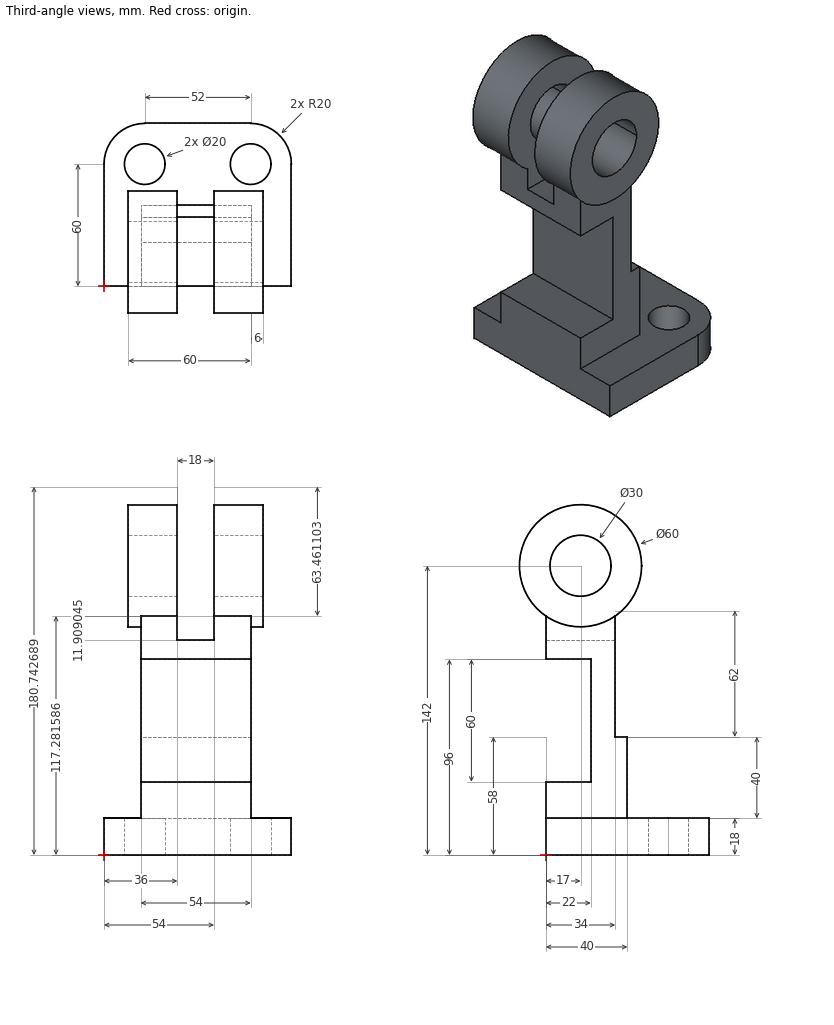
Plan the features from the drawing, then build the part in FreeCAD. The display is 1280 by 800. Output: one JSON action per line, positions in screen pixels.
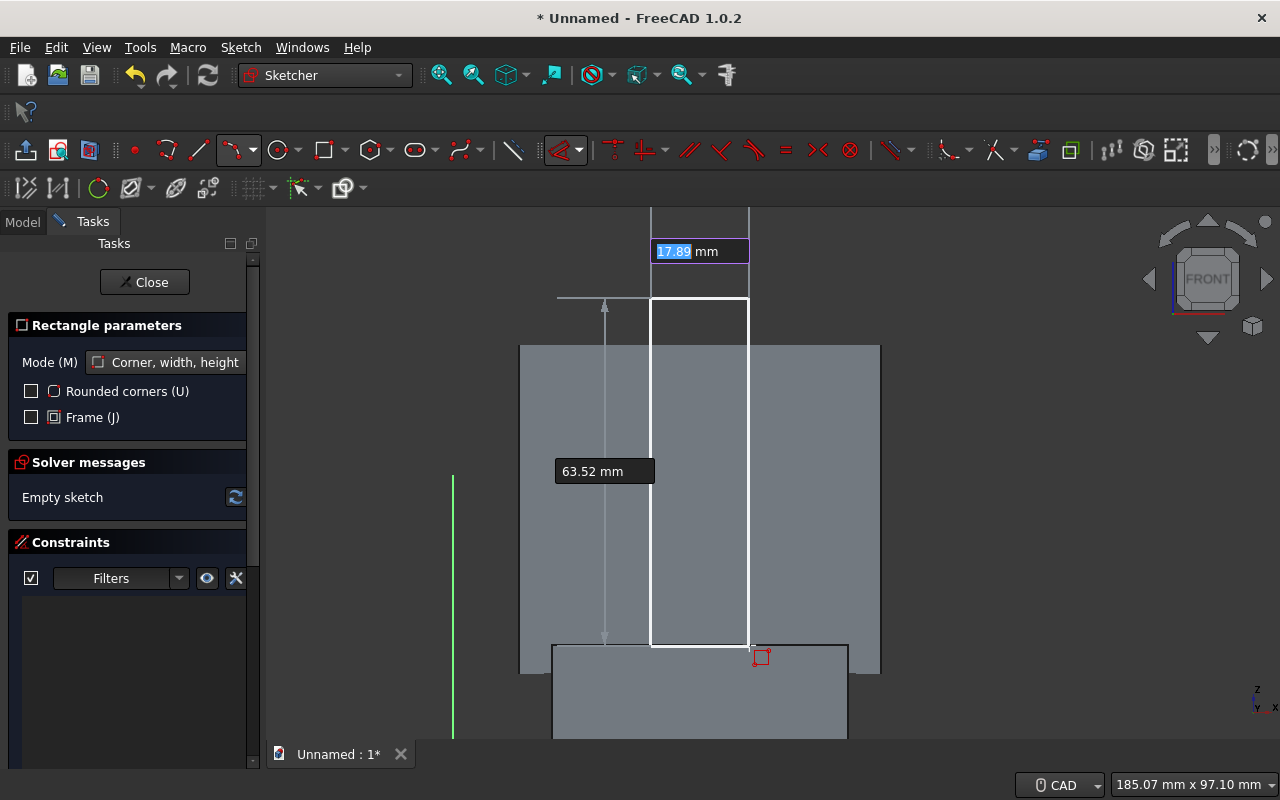
{"action": "type", "text": "18"}
{"action": "key", "text": "Tab"}
{"action": "type", "text": "63.461103"}
{"action": "key", "text": "Return"}
{"action": "key", "text": "Escape"}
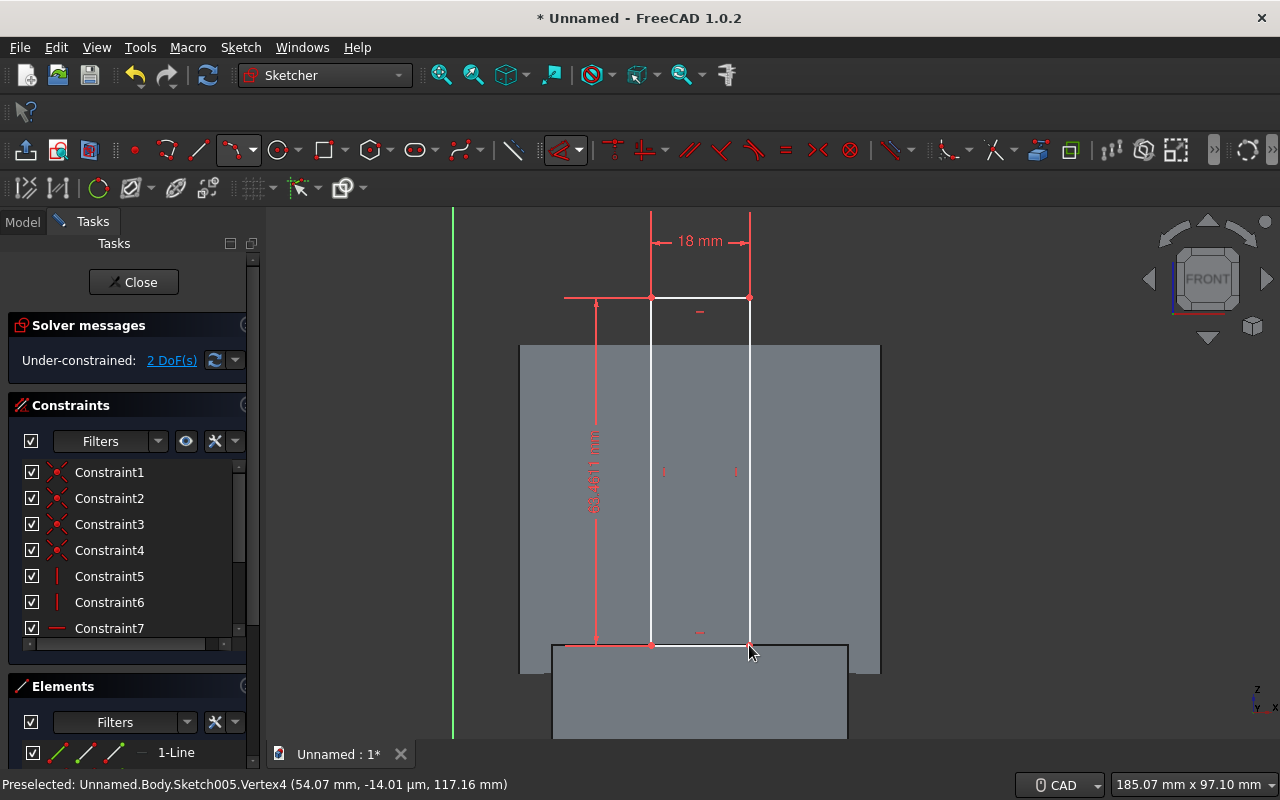
{"action": "left_click", "coordinate": [651, 298]}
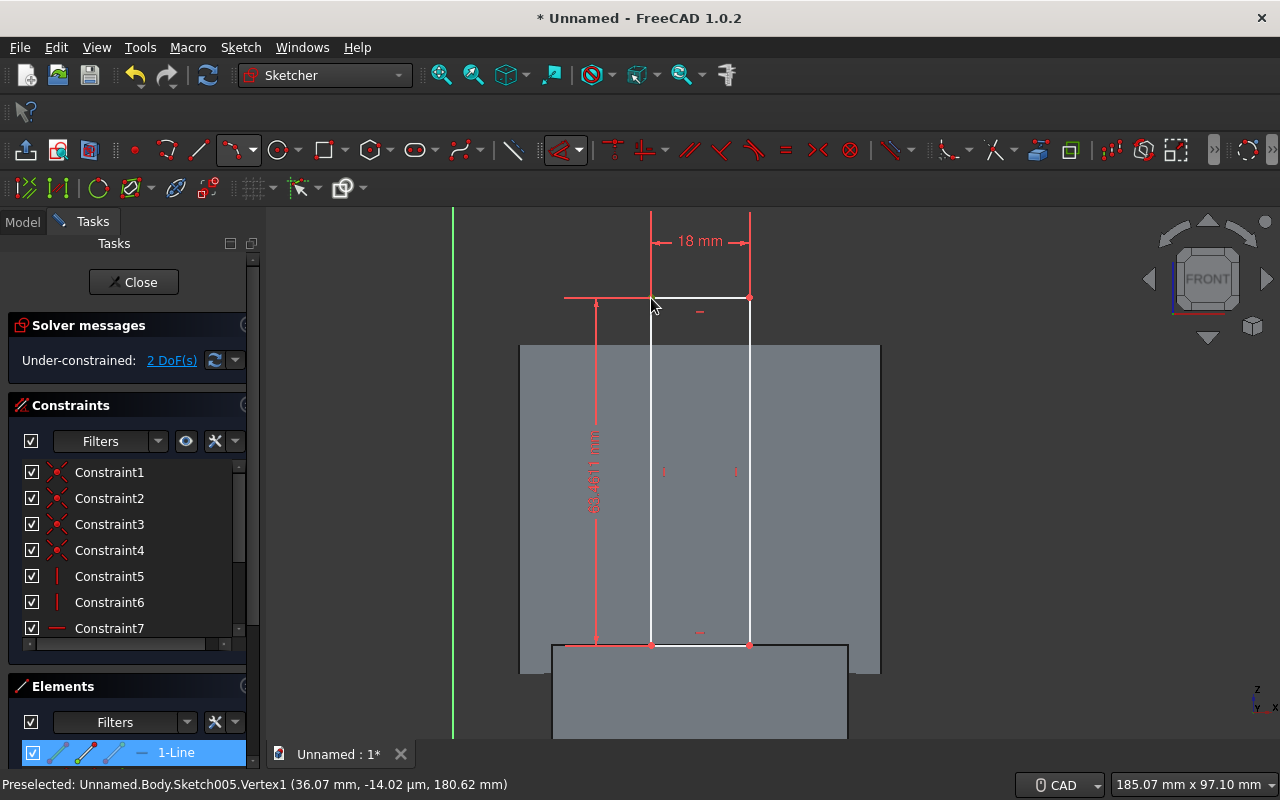
{"action": "left_click", "coordinate": [582, 150]}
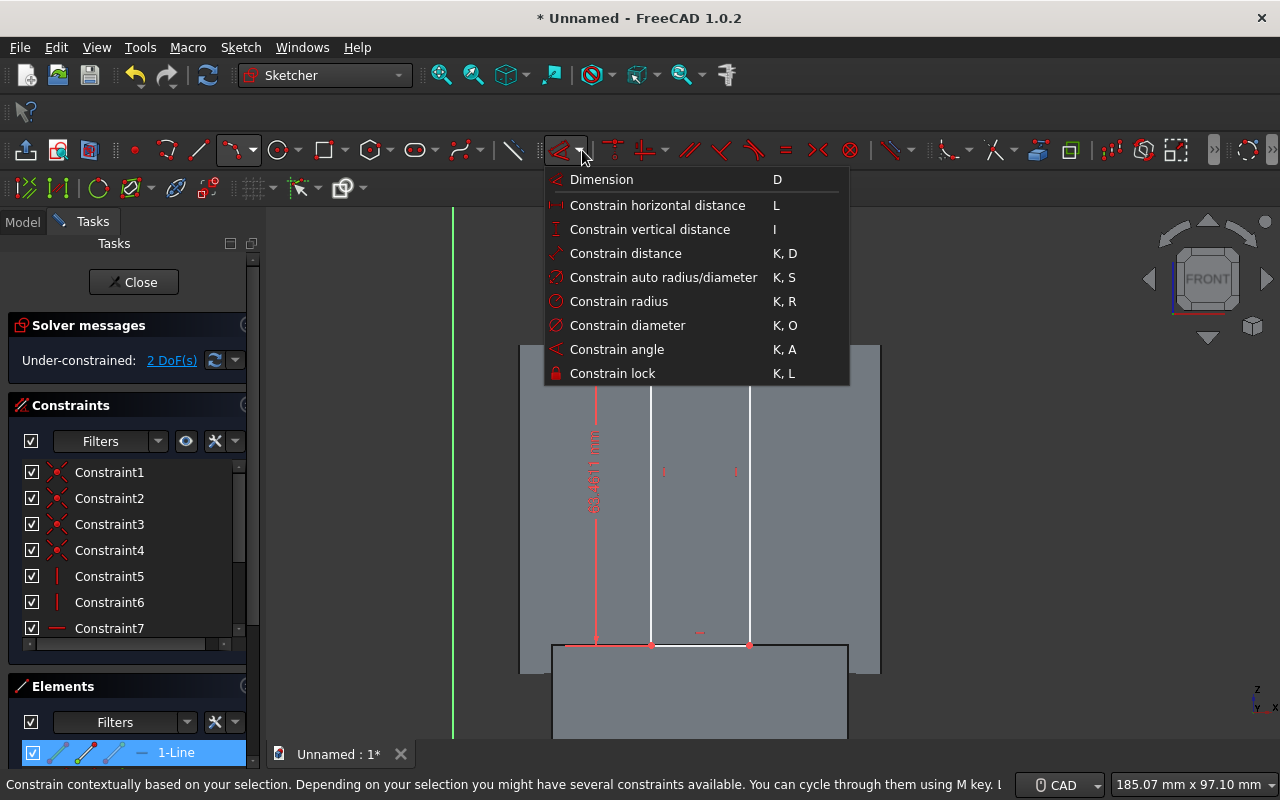
{"action": "left_click", "coordinate": [697, 205]}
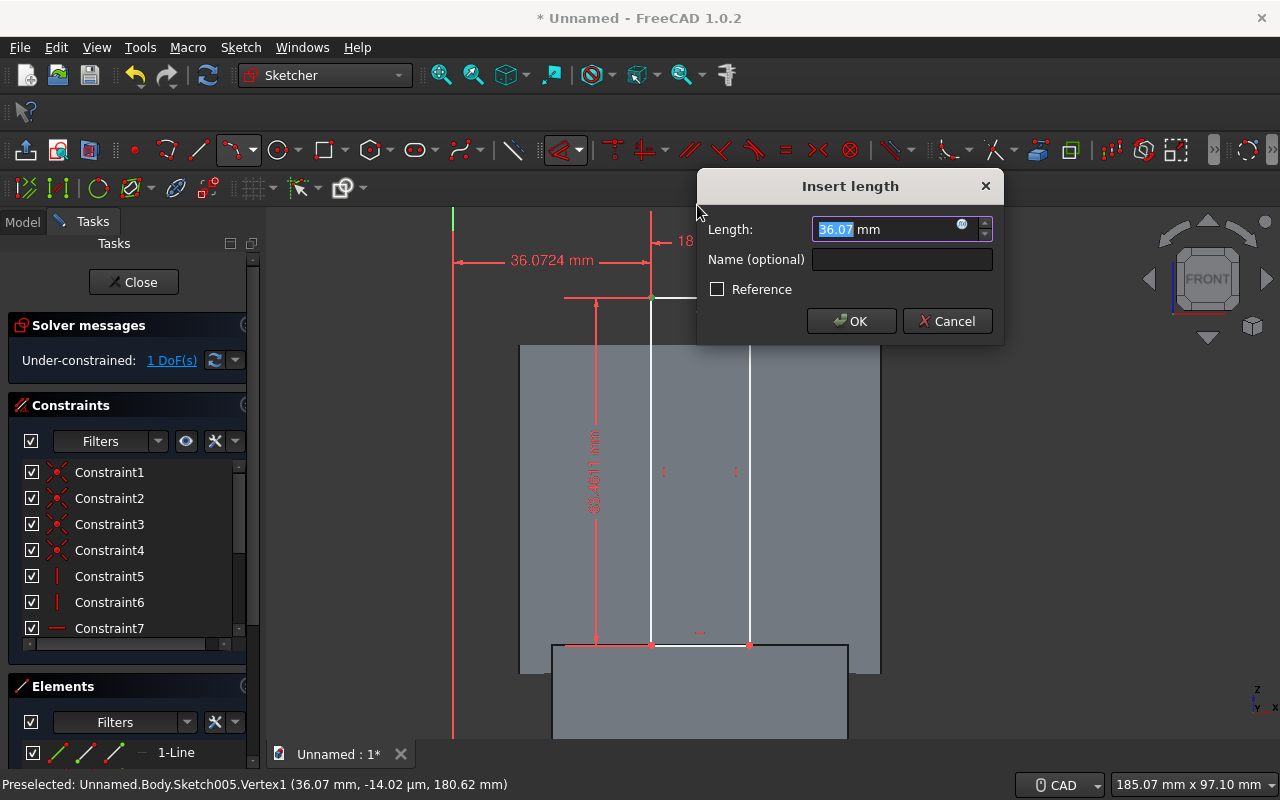
{"action": "type", "text": "36"}
{"action": "key", "text": "Return"}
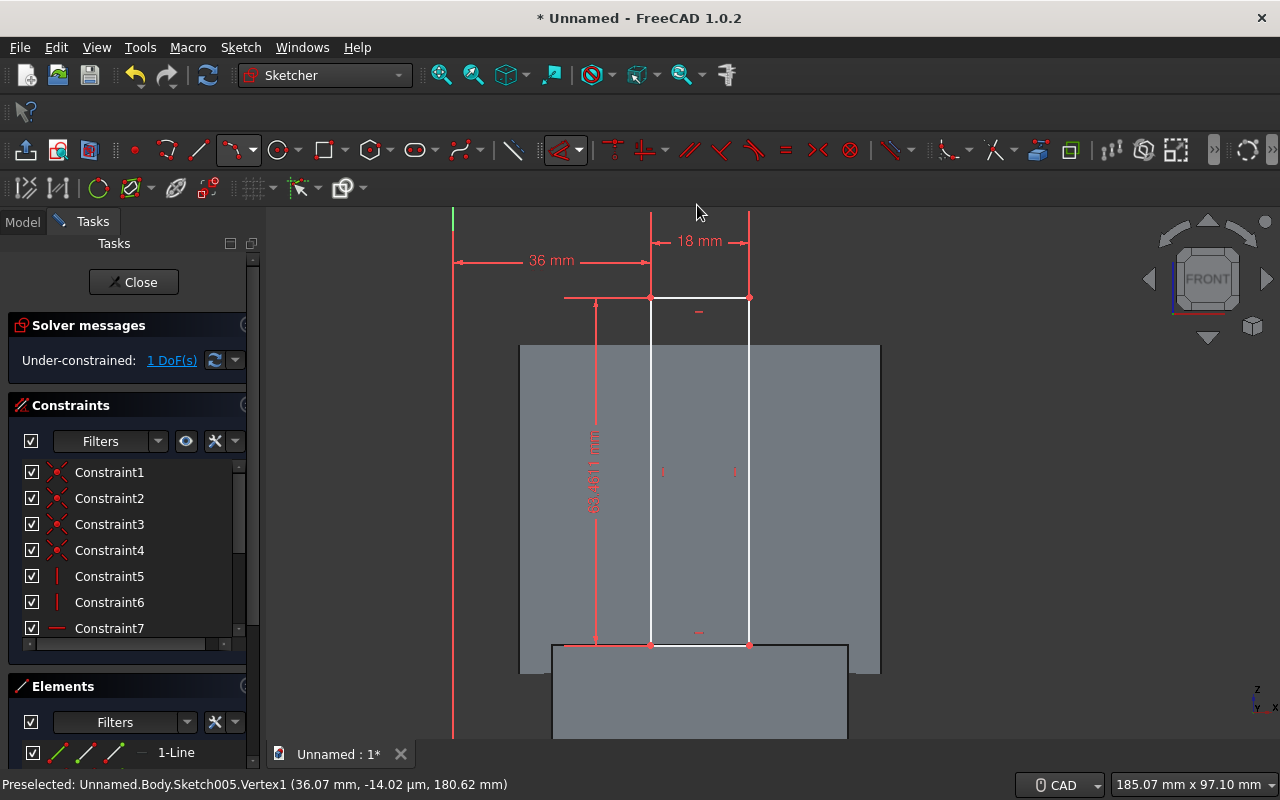
{"action": "left_click", "coordinate": [651, 298]}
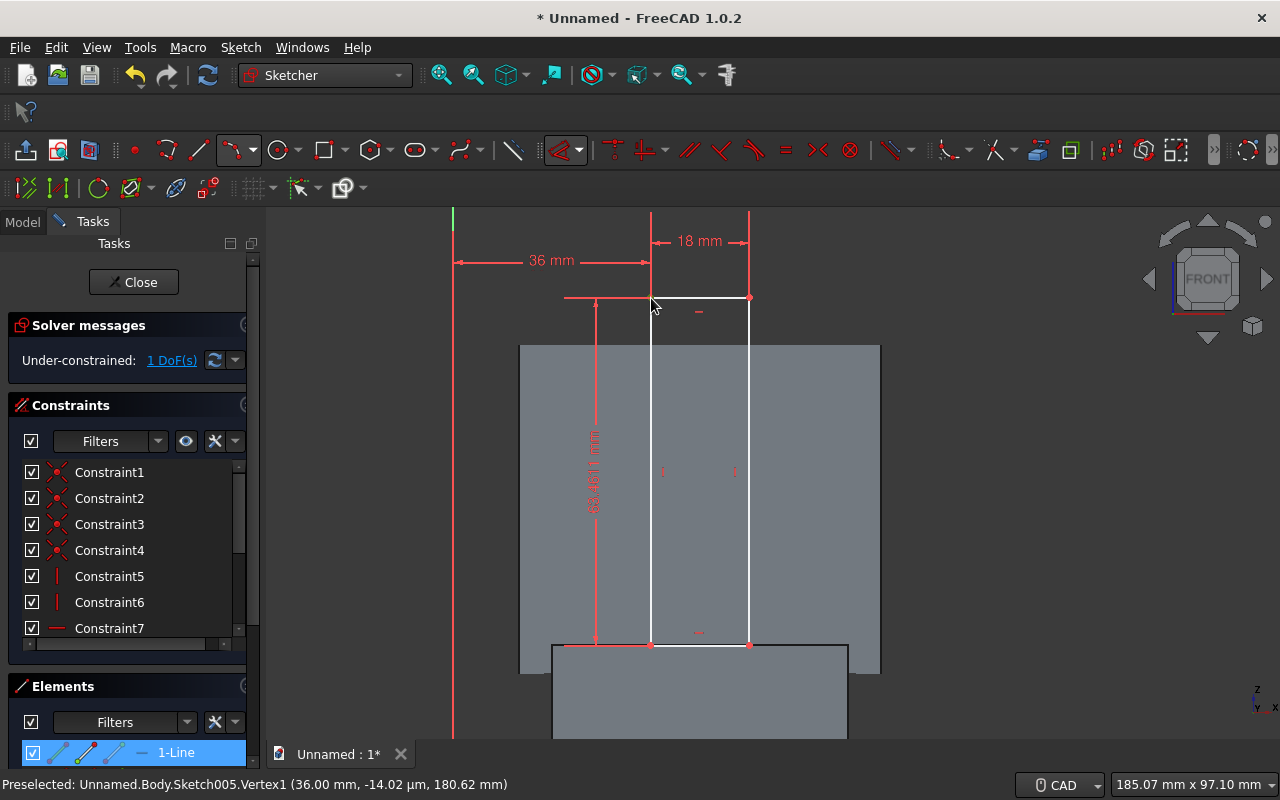
{"action": "left_click", "coordinate": [582, 150]}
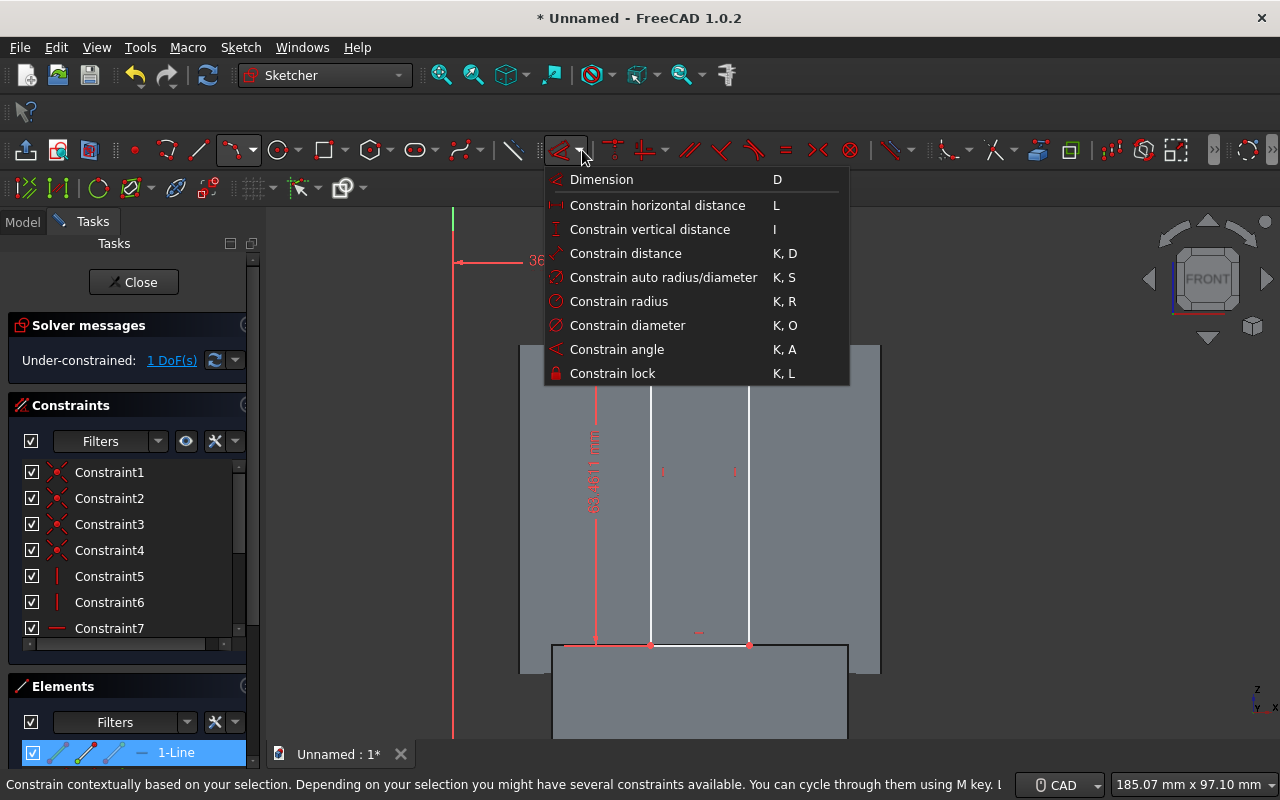
{"action": "left_click", "coordinate": [697, 229]}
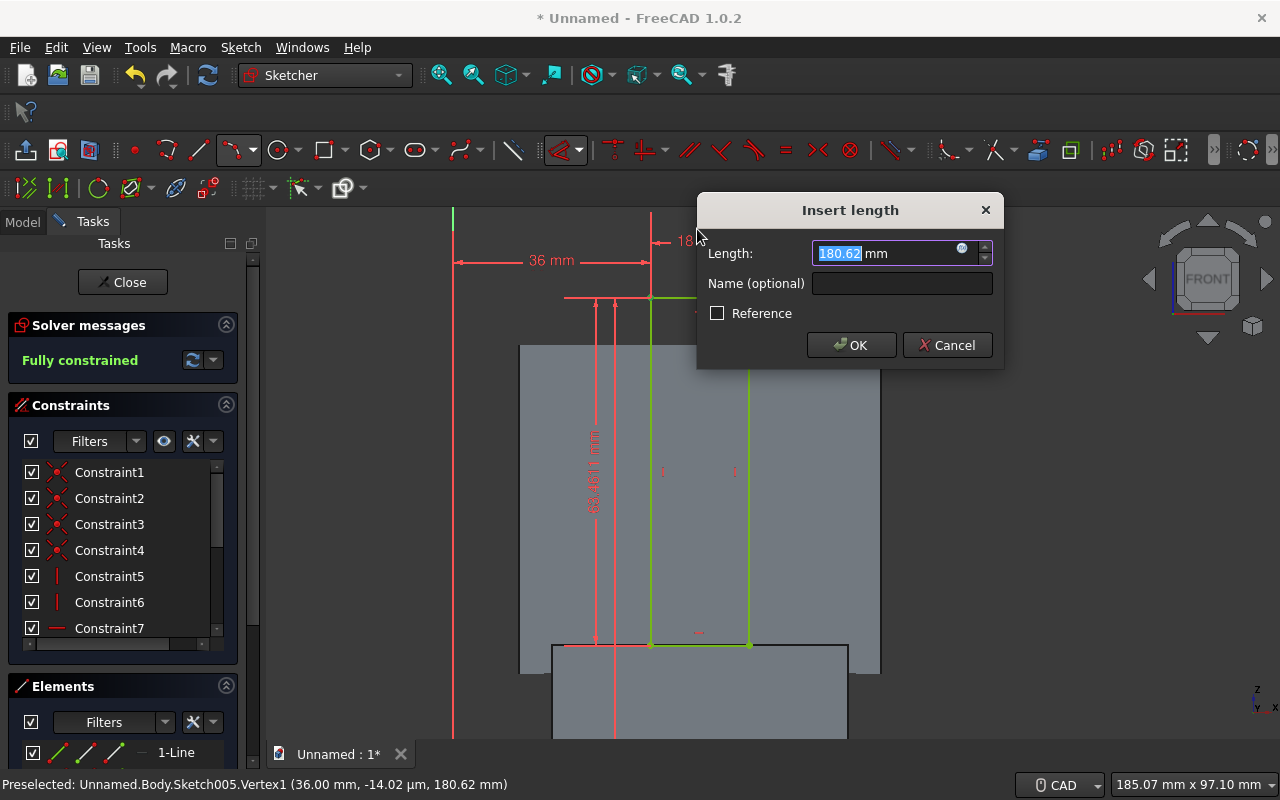
{"action": "type", "text": "180.742689"}
{"action": "key", "text": "Return"}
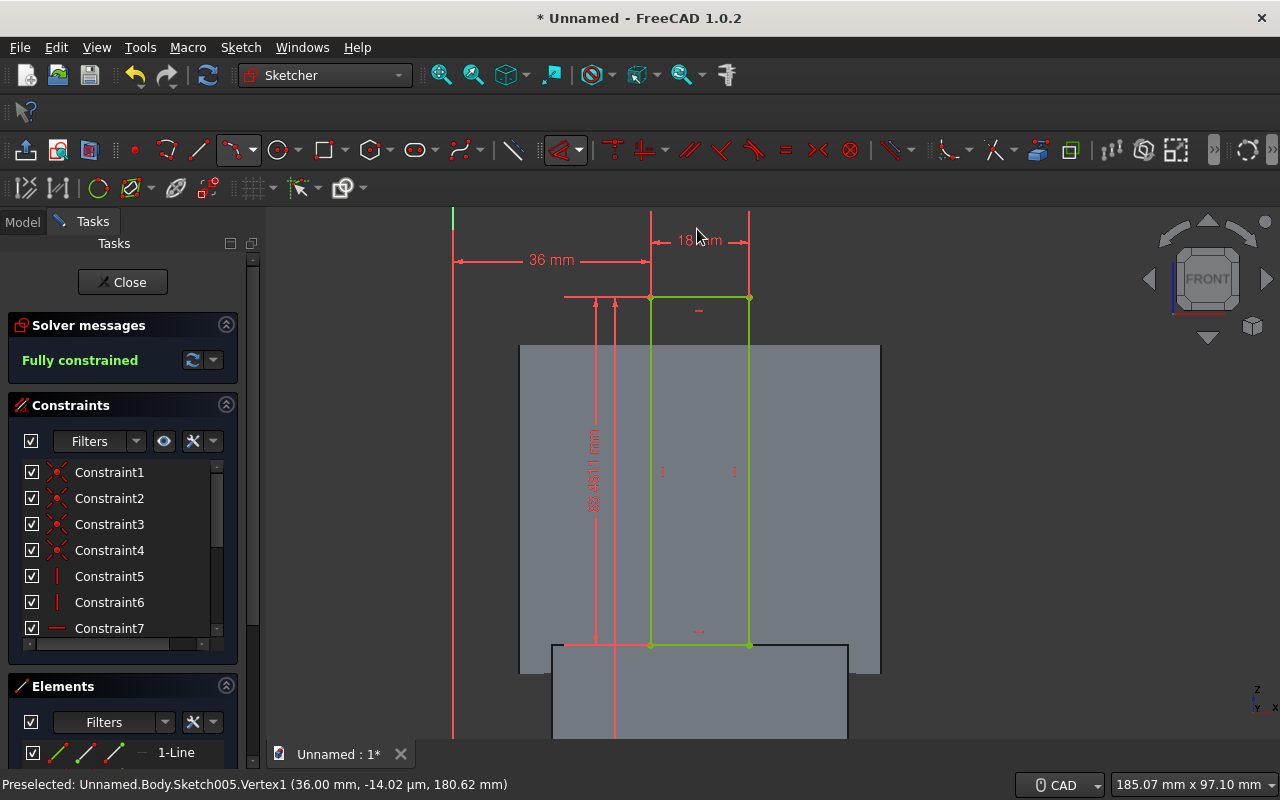
{"action": "left_click", "coordinate": [123, 282]}